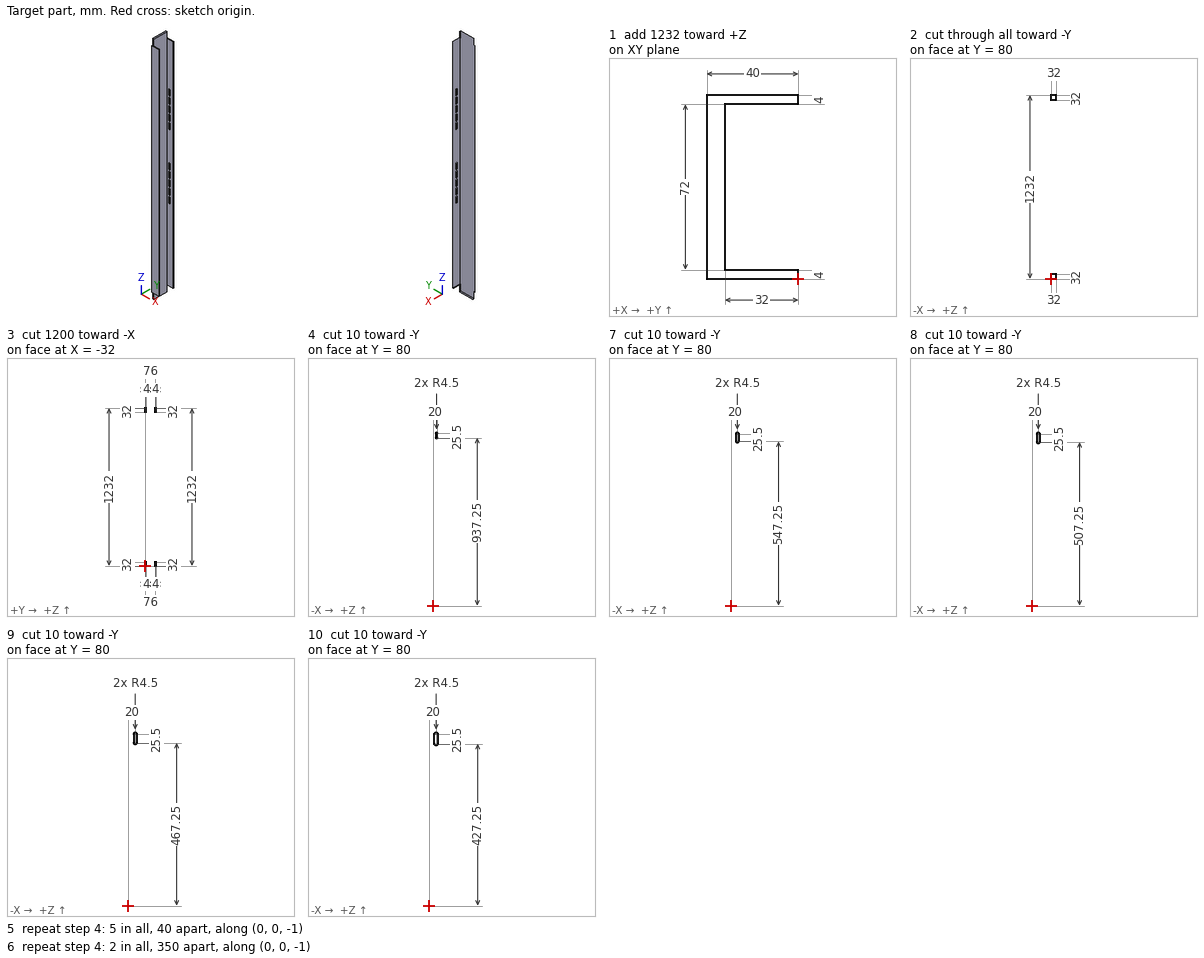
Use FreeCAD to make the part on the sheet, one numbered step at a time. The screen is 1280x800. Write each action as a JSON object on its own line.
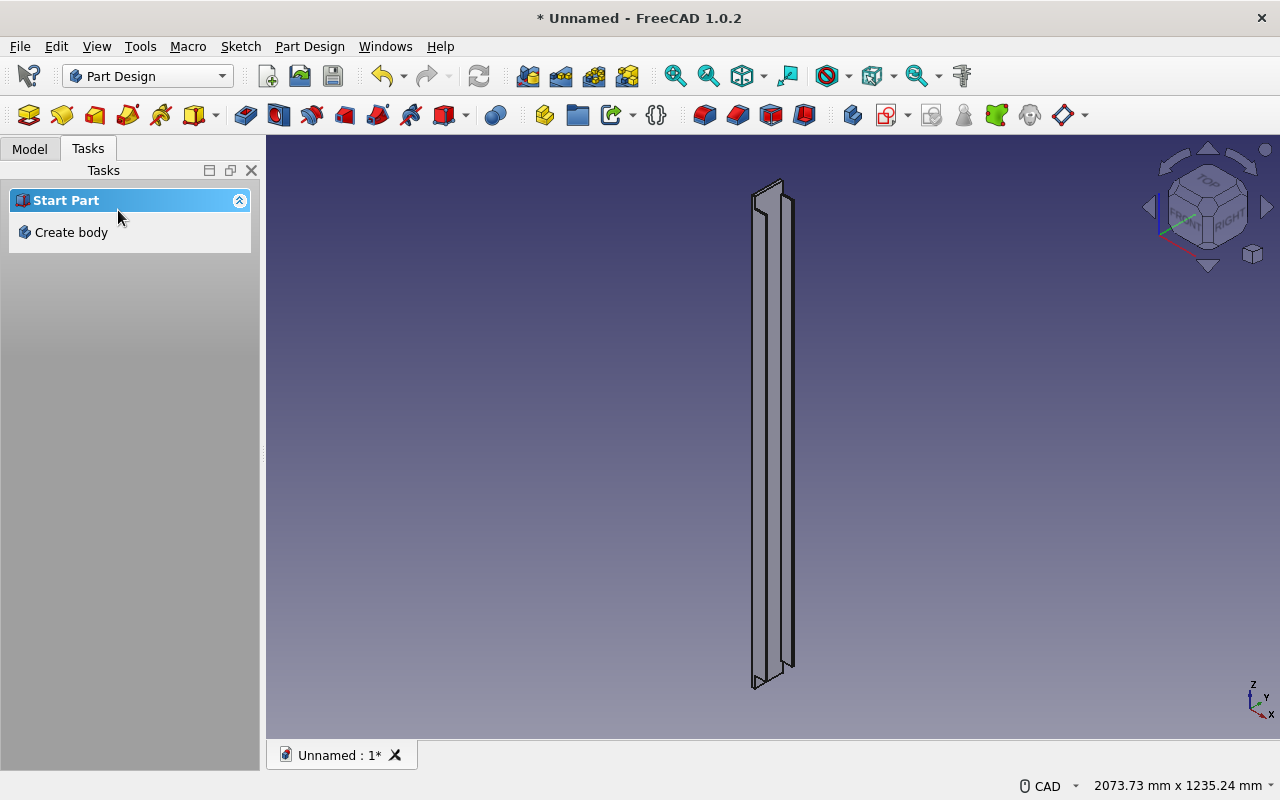
{"action": "key", "text": "3"}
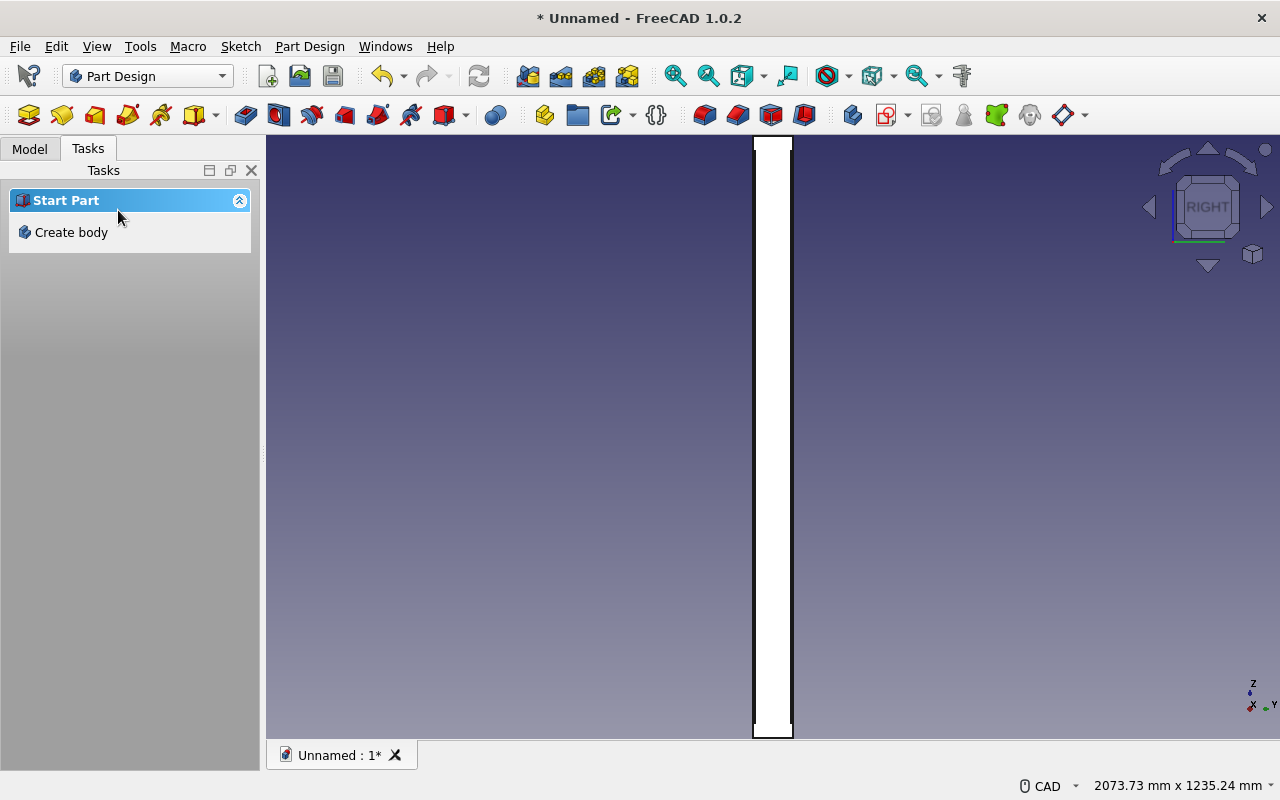
{"action": "left_click", "coordinate": [773, 178]}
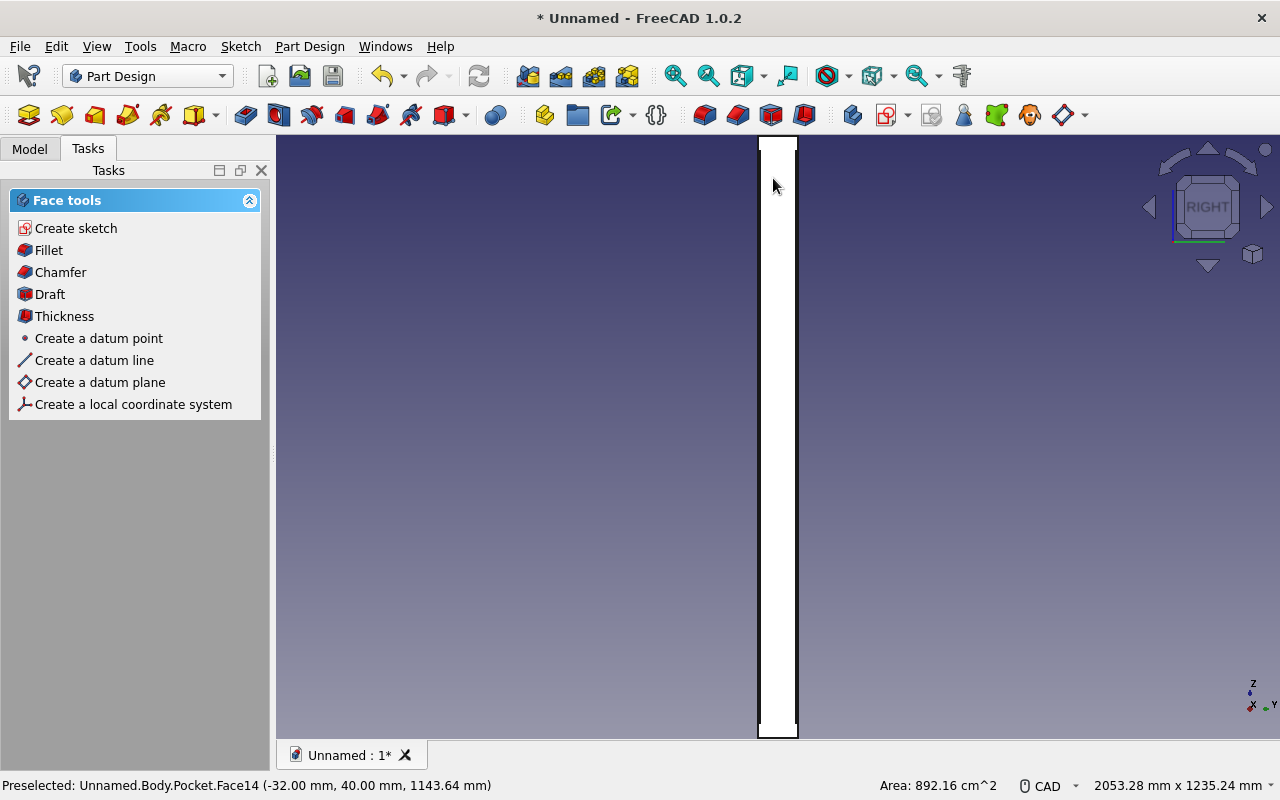
{"action": "left_click", "coordinate": [886, 116]}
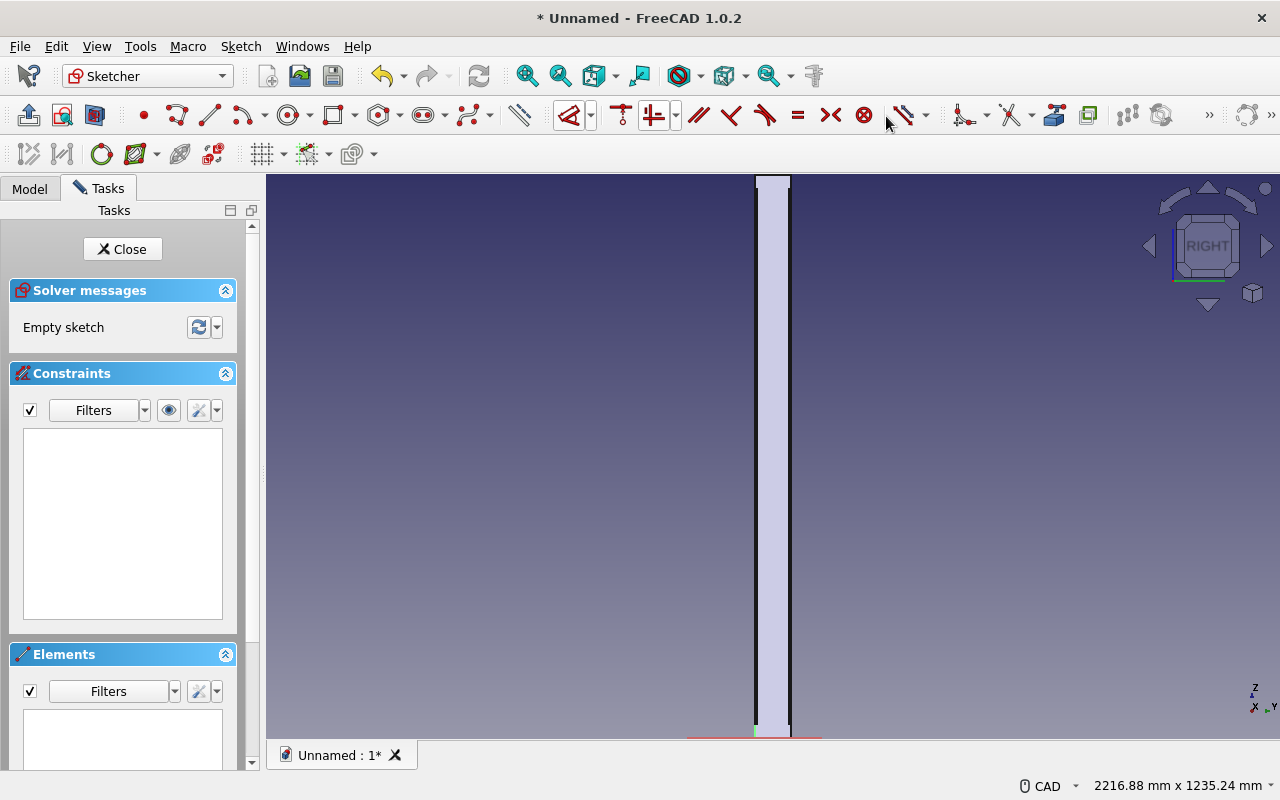
{"action": "left_click", "coordinate": [95, 116]}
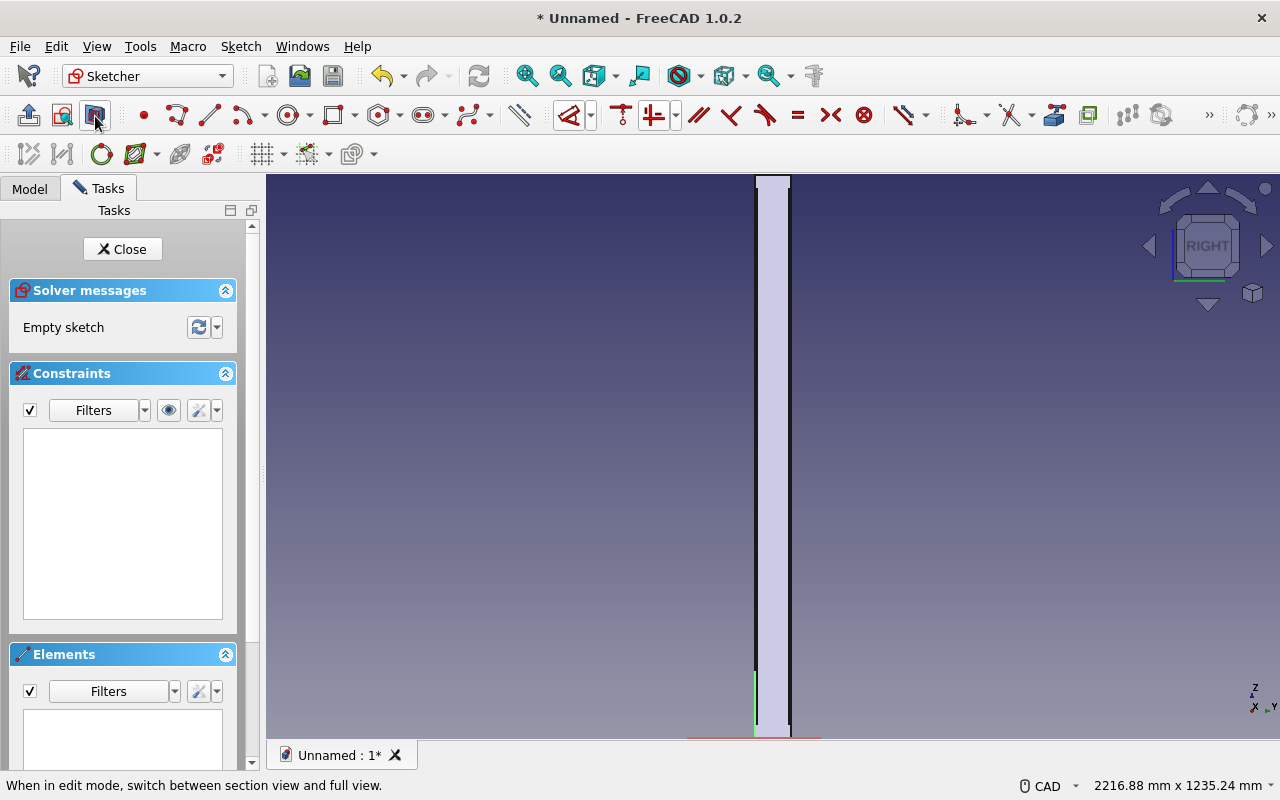
{"action": "scroll", "coordinate": [565, 457], "scroll_direction": "down", "scroll_amount": 2}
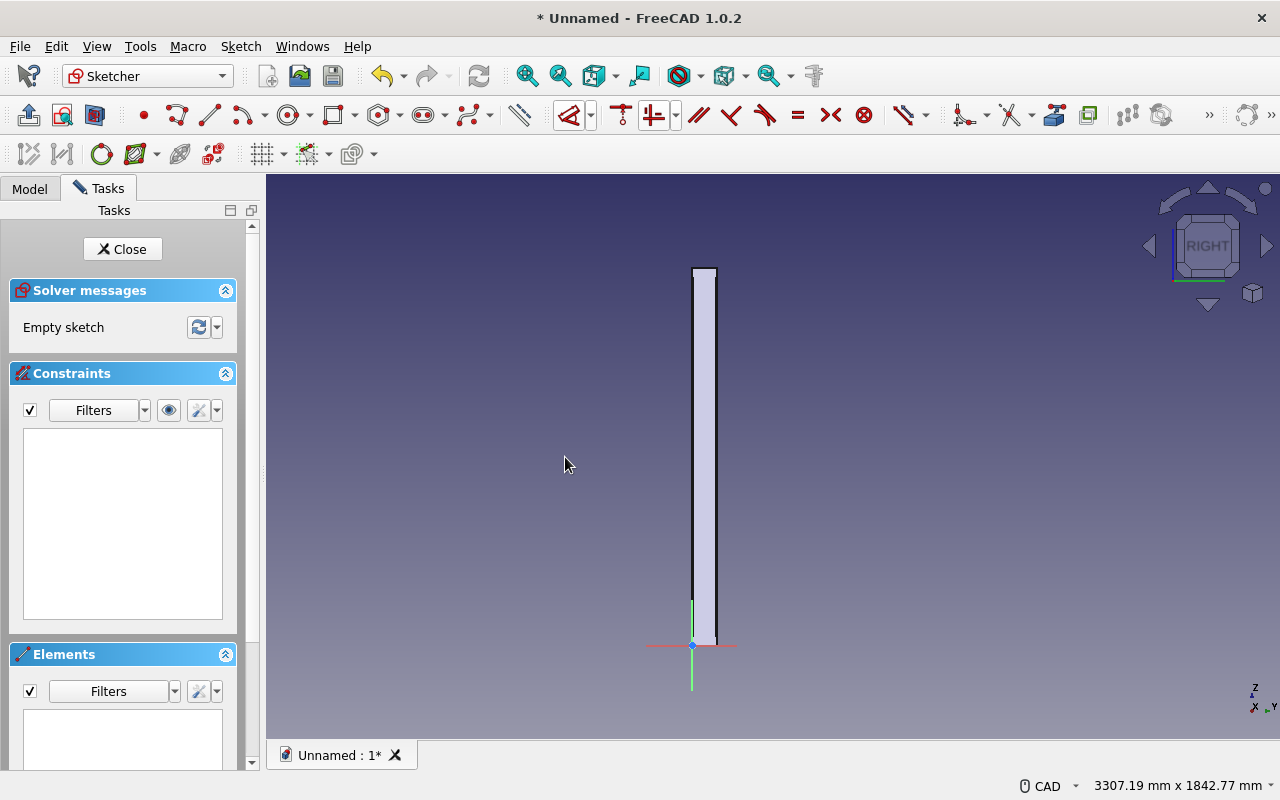
{"action": "left_click", "coordinate": [332, 116]}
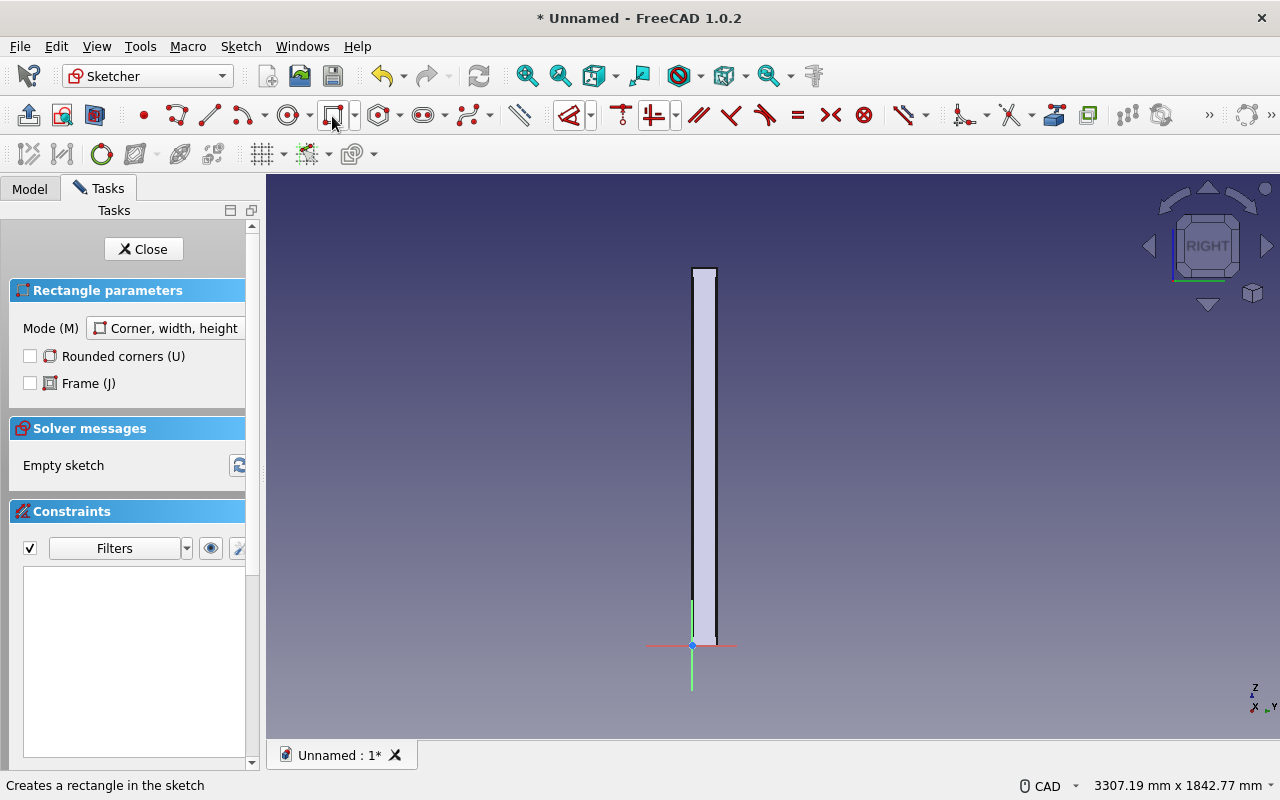
{"action": "scroll", "coordinate": [716, 268], "scroll_direction": "up", "scroll_amount": 13}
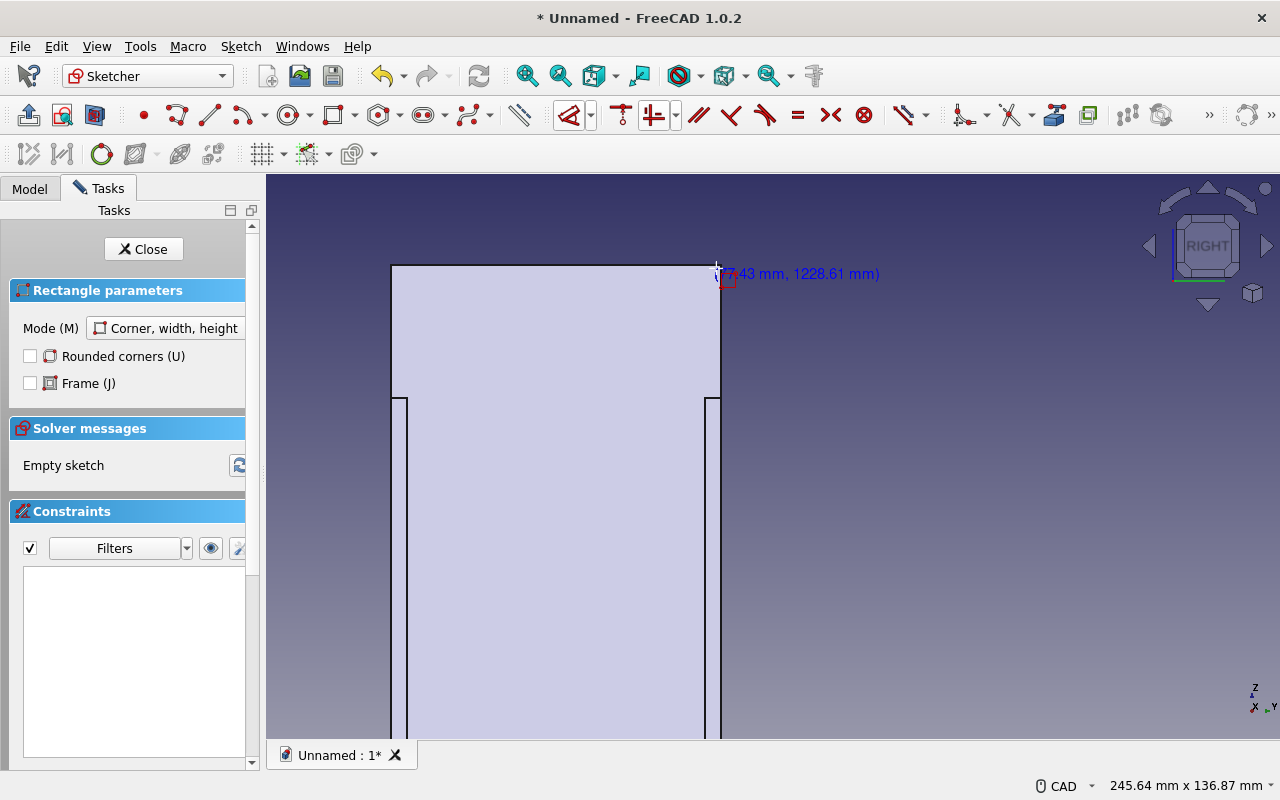
{"action": "scroll", "coordinate": [716, 268], "scroll_direction": "down", "scroll_amount": 13}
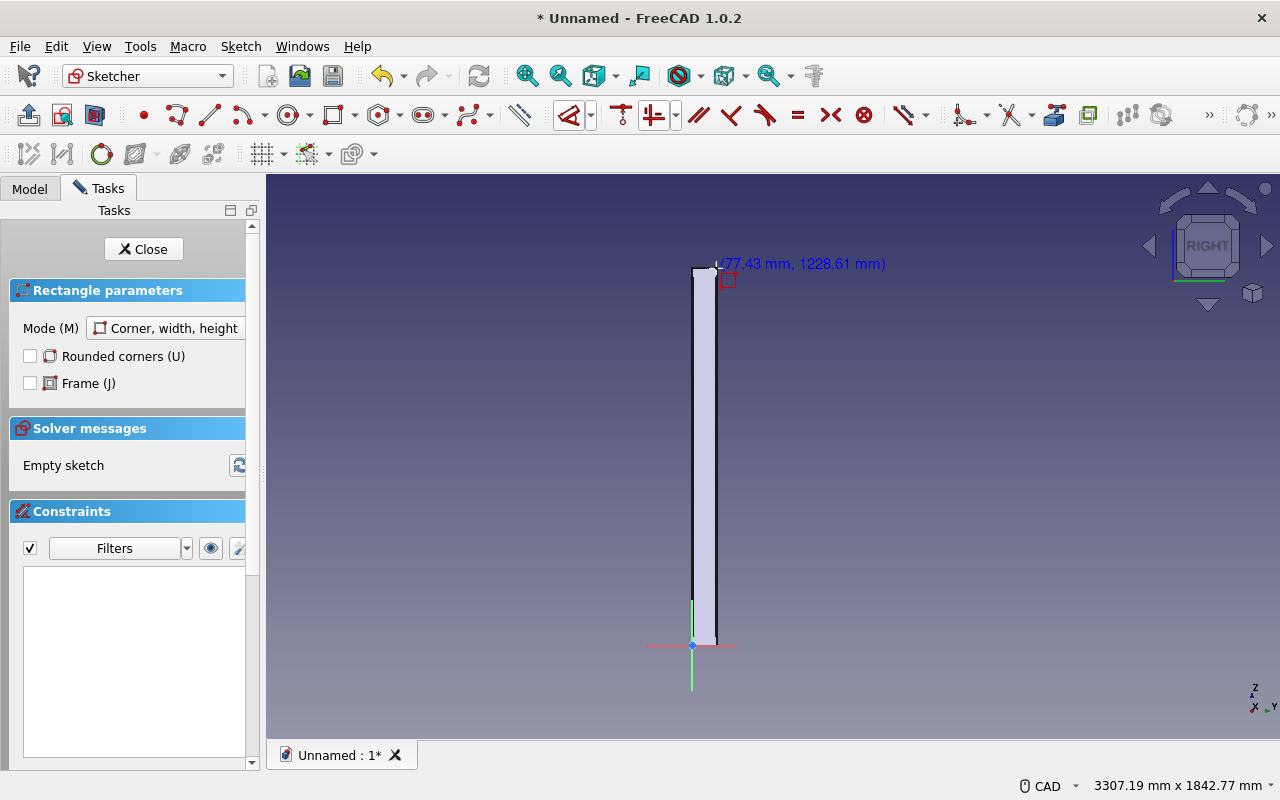
{"action": "left_click", "coordinate": [716, 268]}
{"action": "mouse_move", "coordinate": [717, 278]}